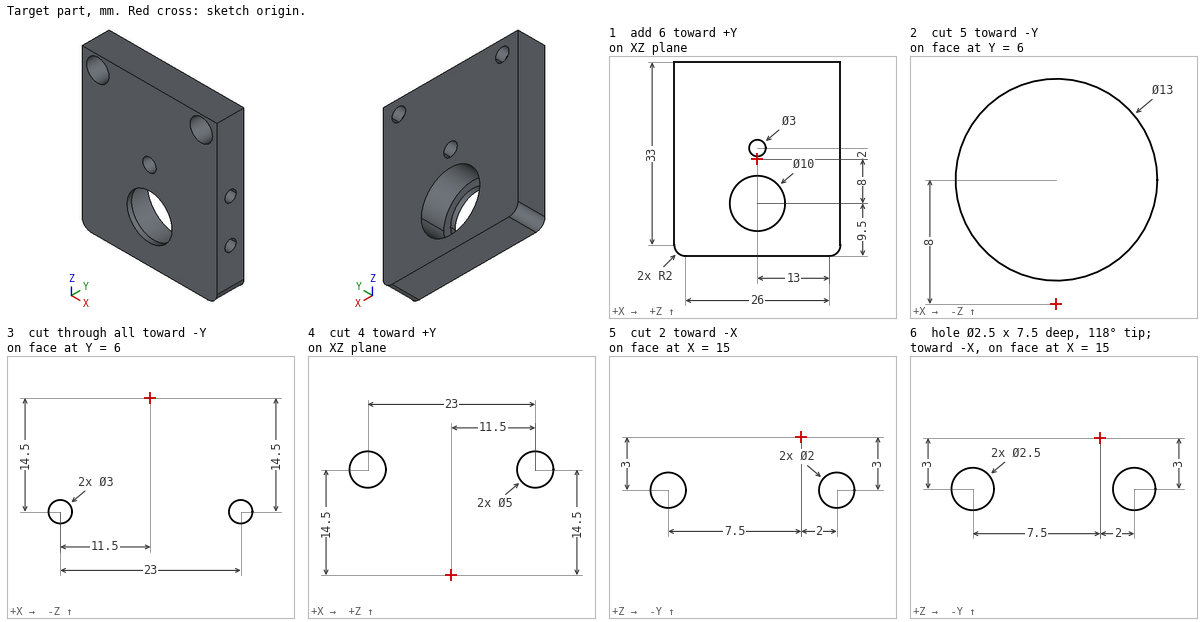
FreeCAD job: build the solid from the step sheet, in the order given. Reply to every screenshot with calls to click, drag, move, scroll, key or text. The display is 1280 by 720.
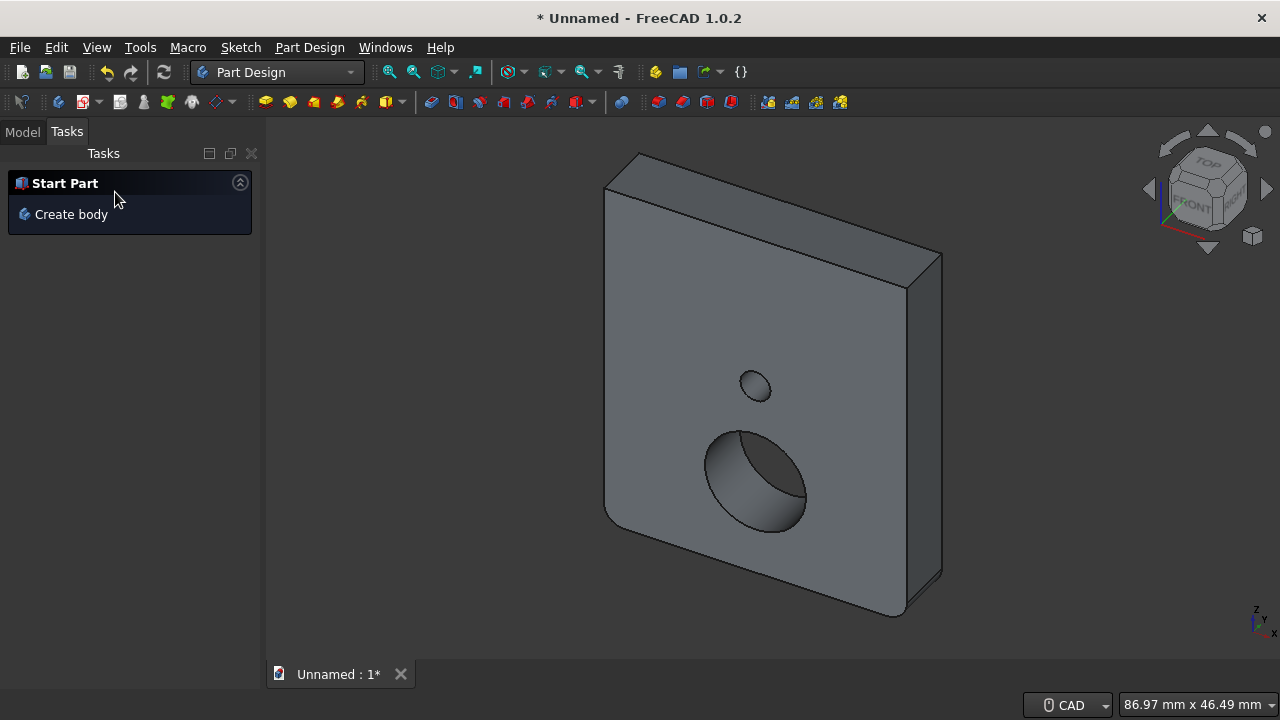
key(4)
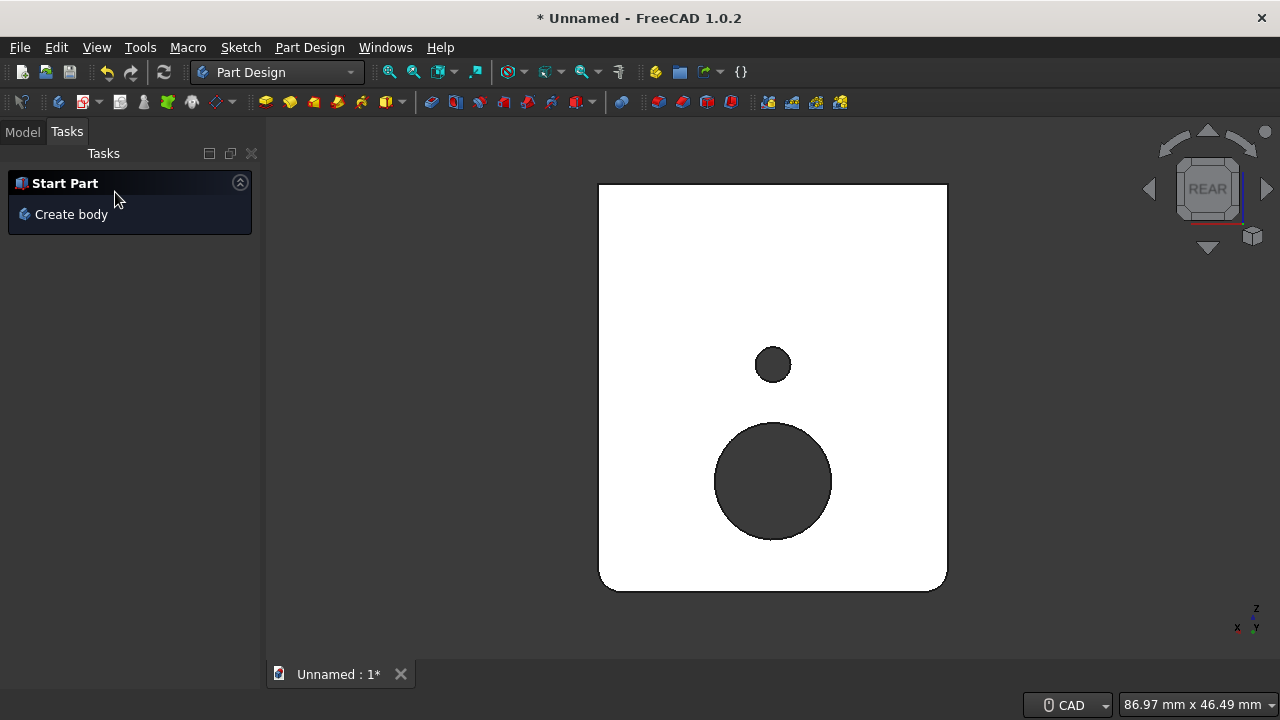
click(723, 270)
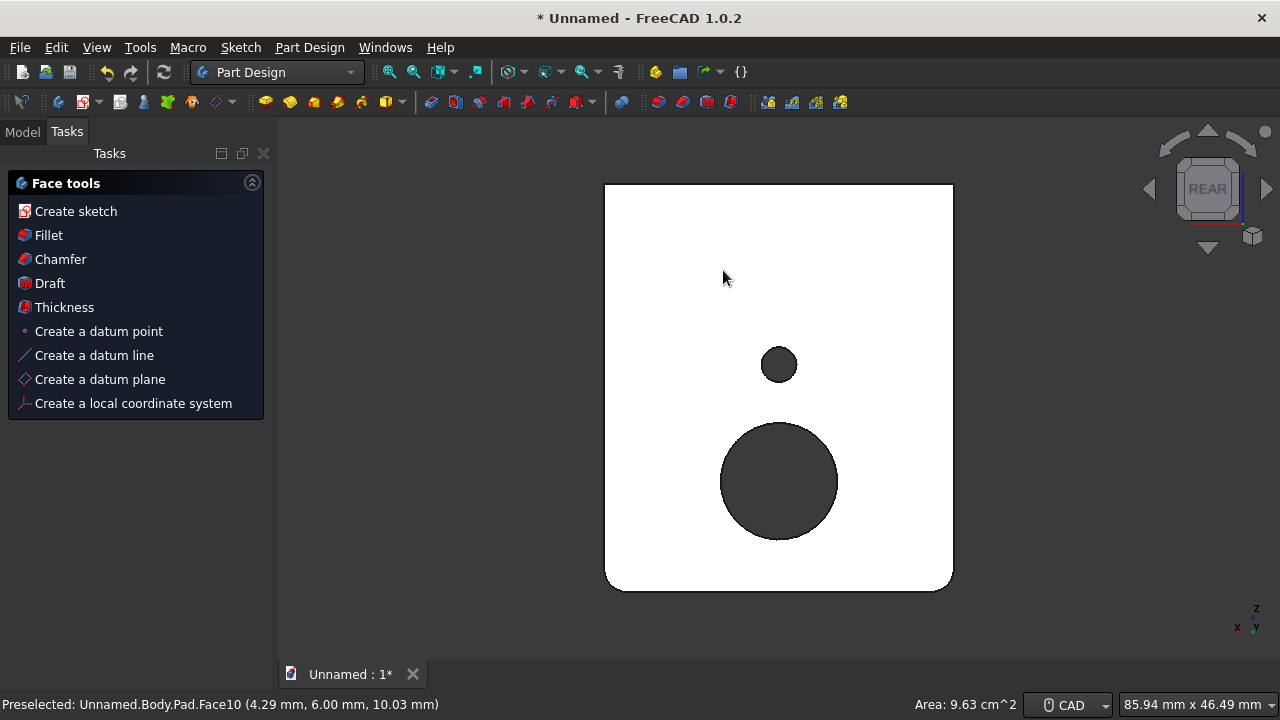
click(84, 102)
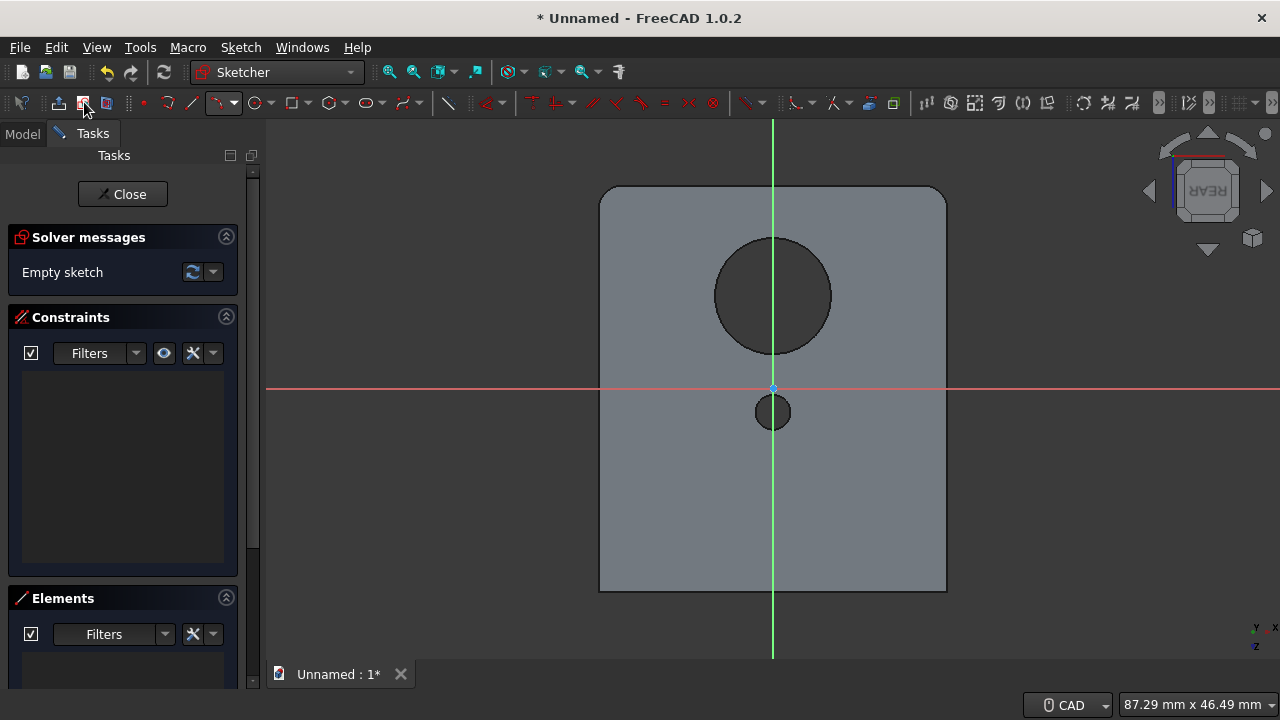
scroll(829, 236, up, 4)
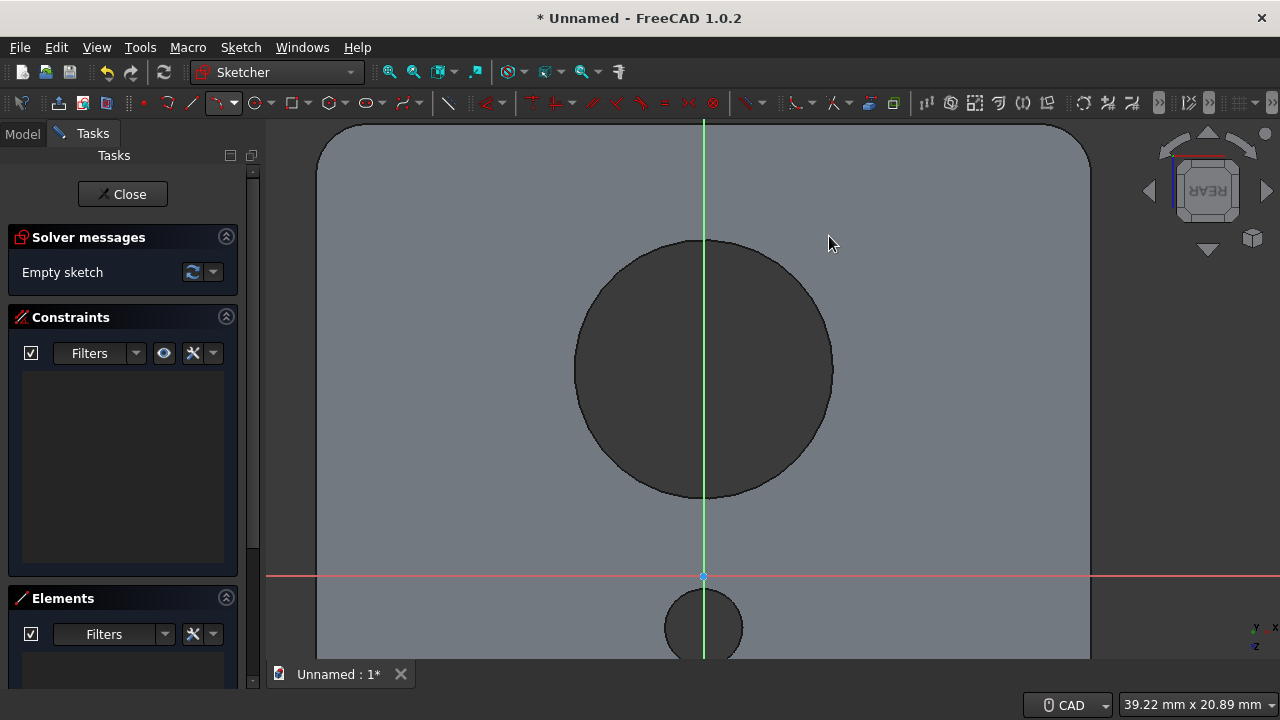
key(g)
key(c)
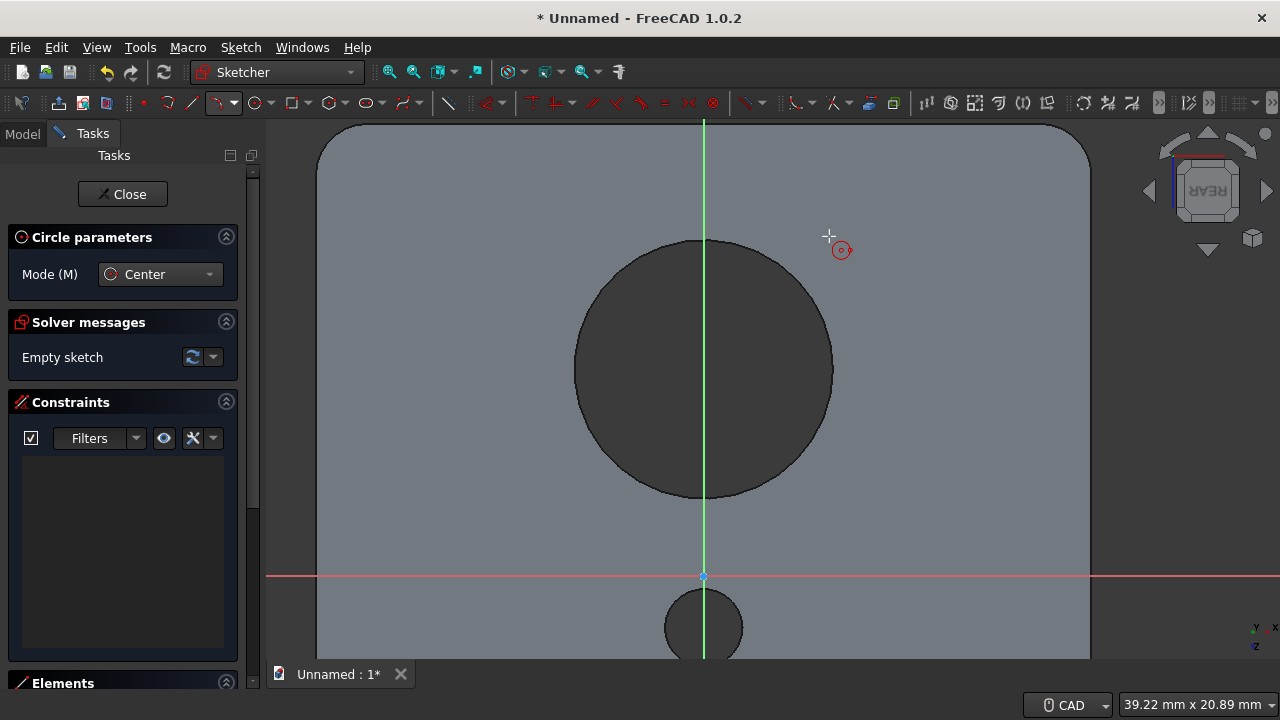
click(704, 369)
click(823, 251)
key(Escape)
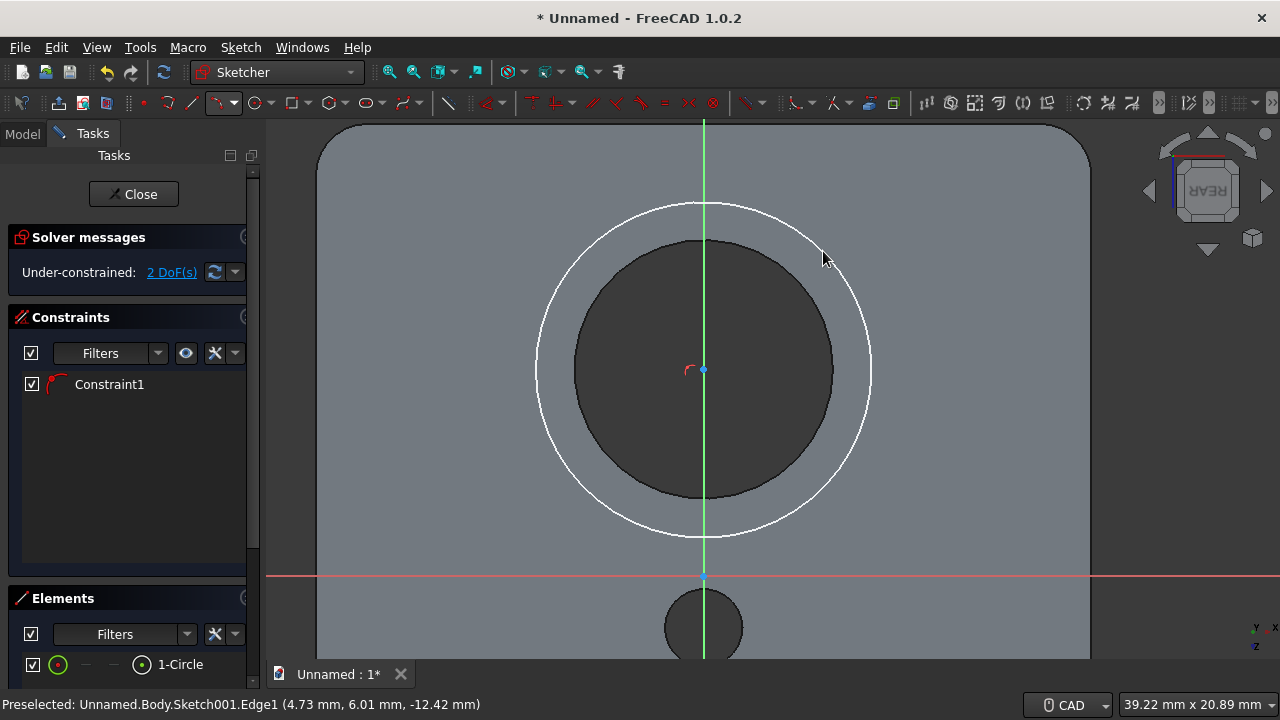
click(486, 104)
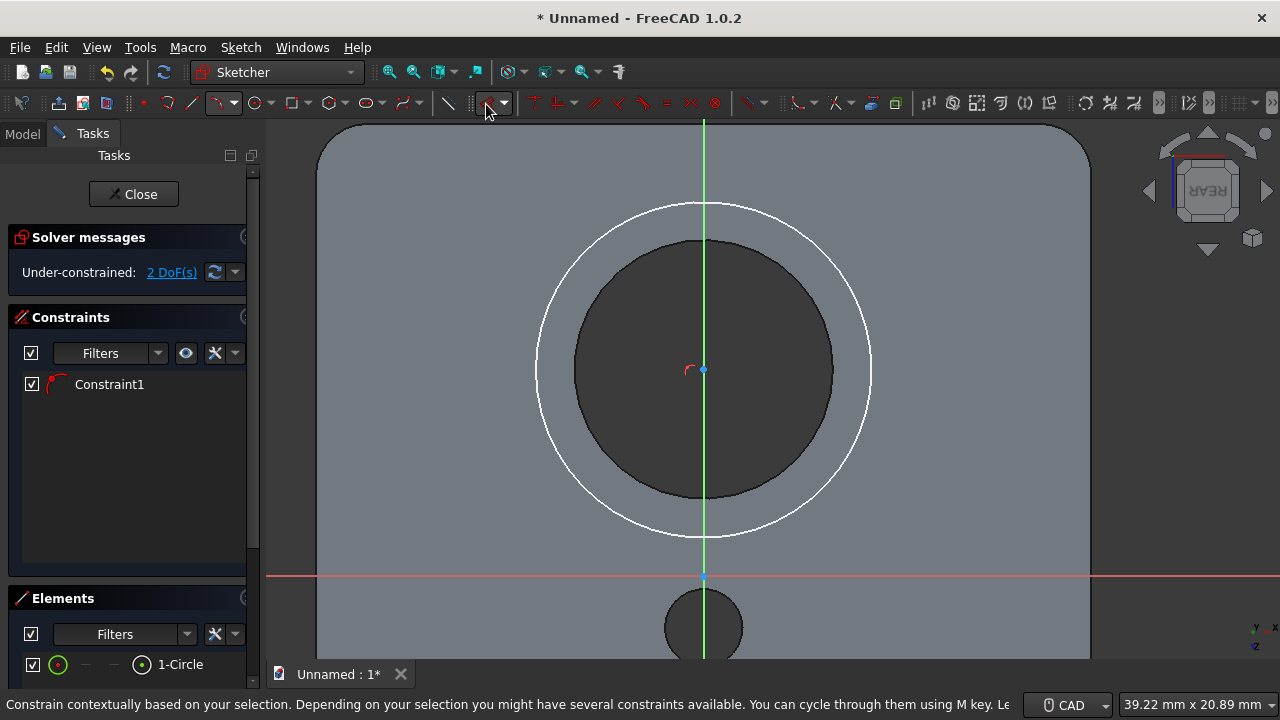
click(822, 251)
click(845, 228)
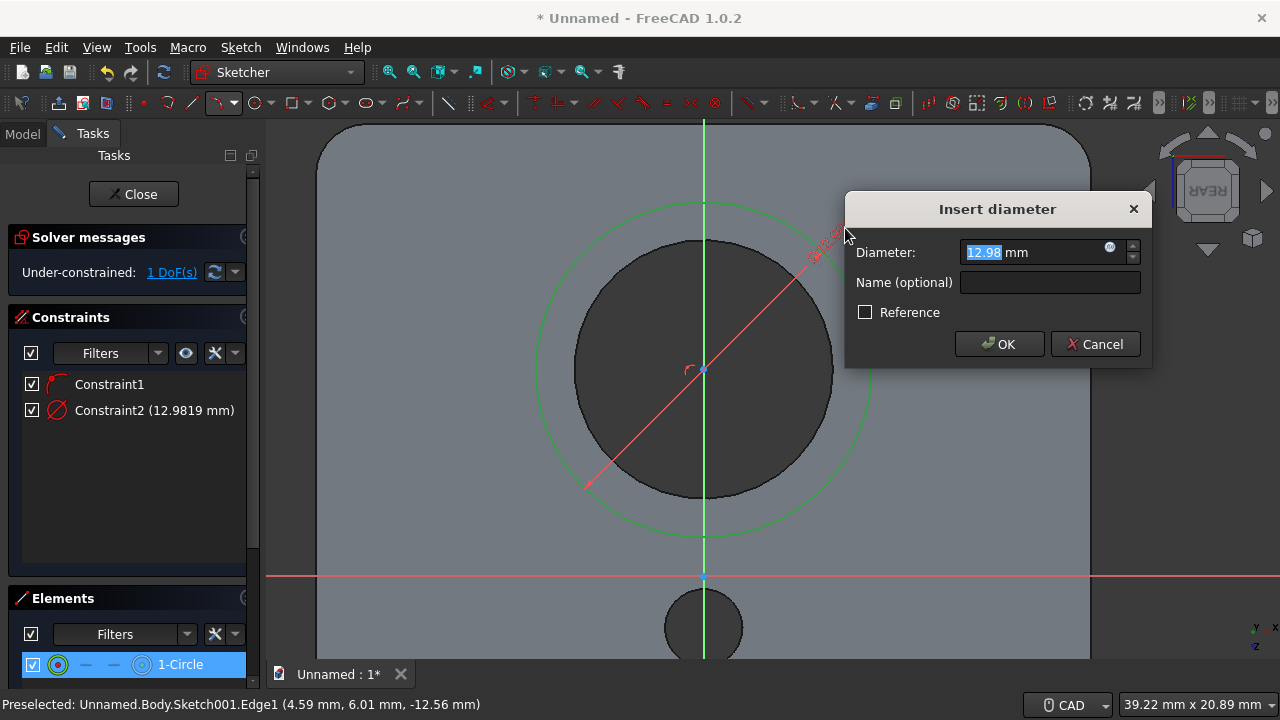
text(13)
key(Return)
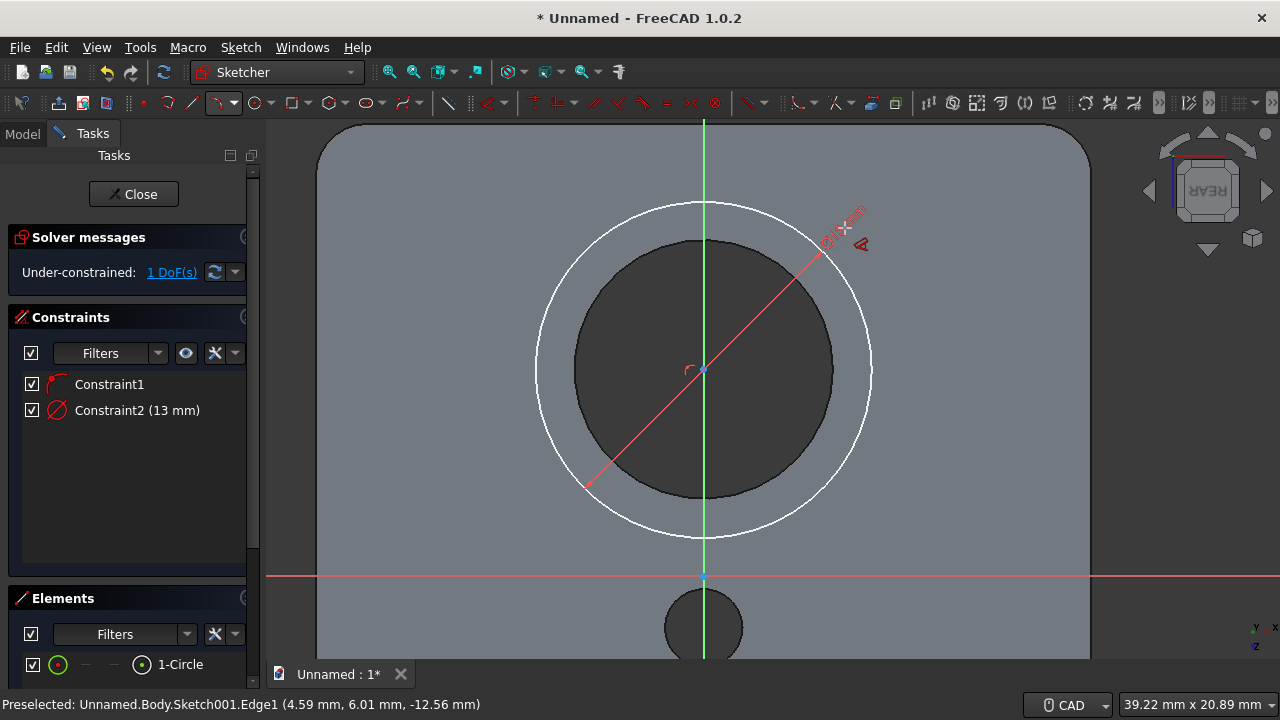
click(704, 370)
click(738, 473)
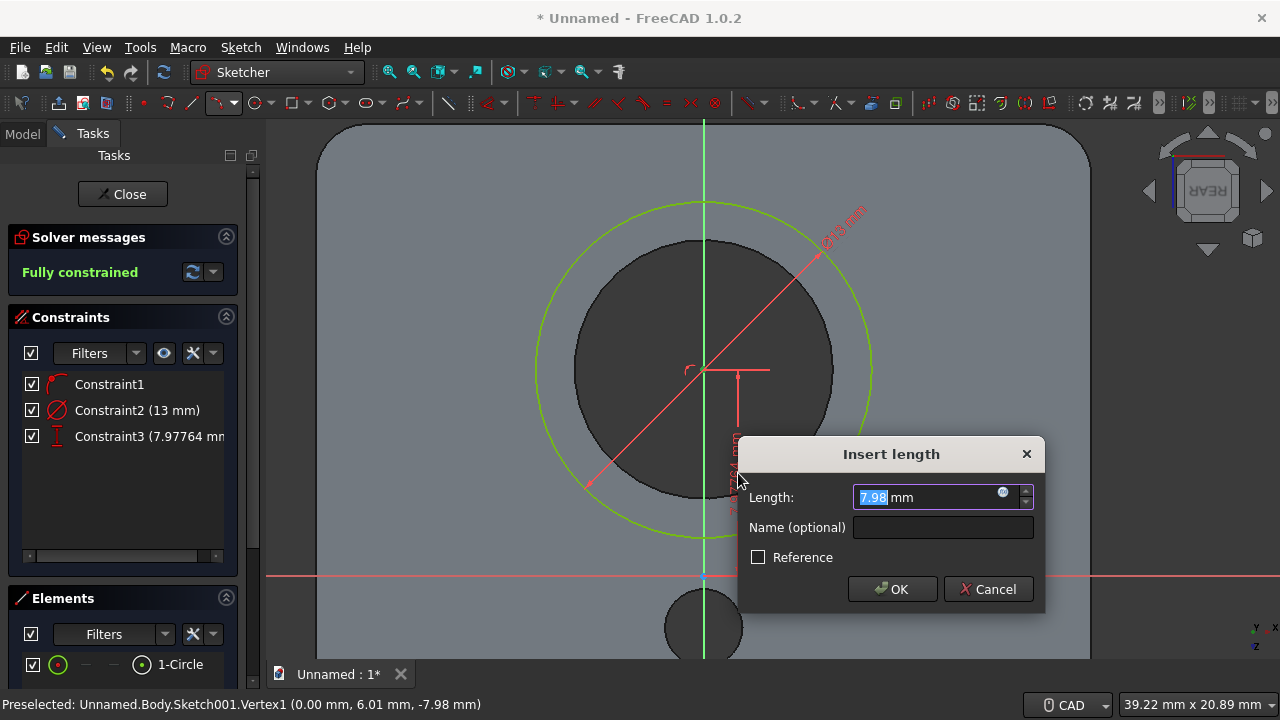
text(8)
key(Return)
key(Escape)